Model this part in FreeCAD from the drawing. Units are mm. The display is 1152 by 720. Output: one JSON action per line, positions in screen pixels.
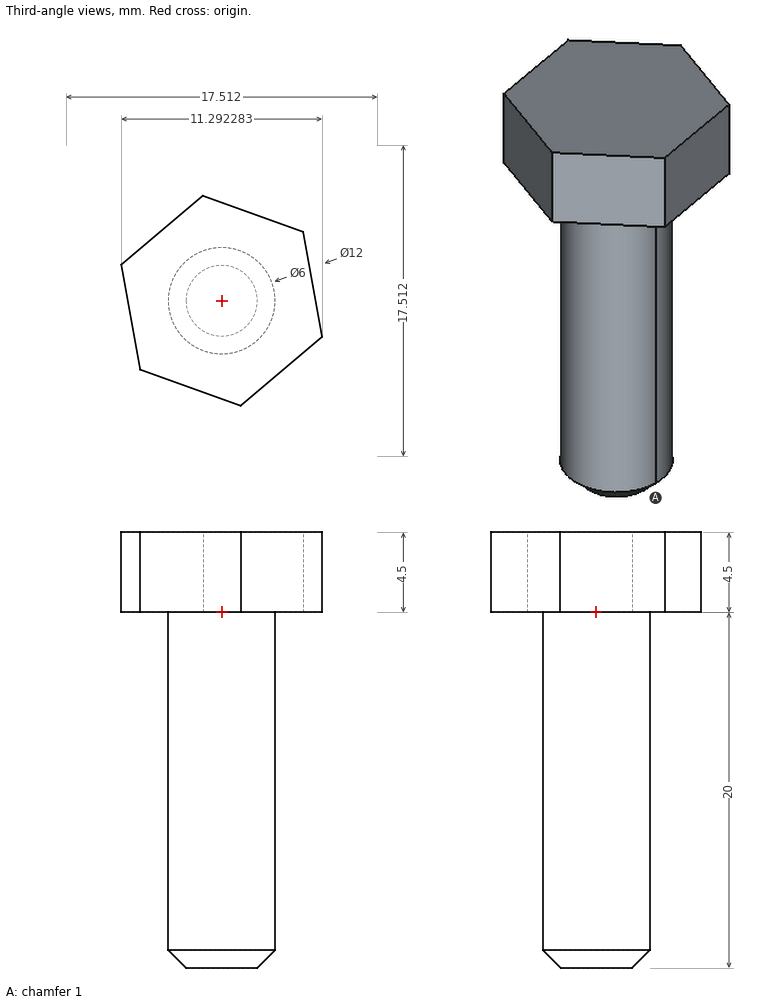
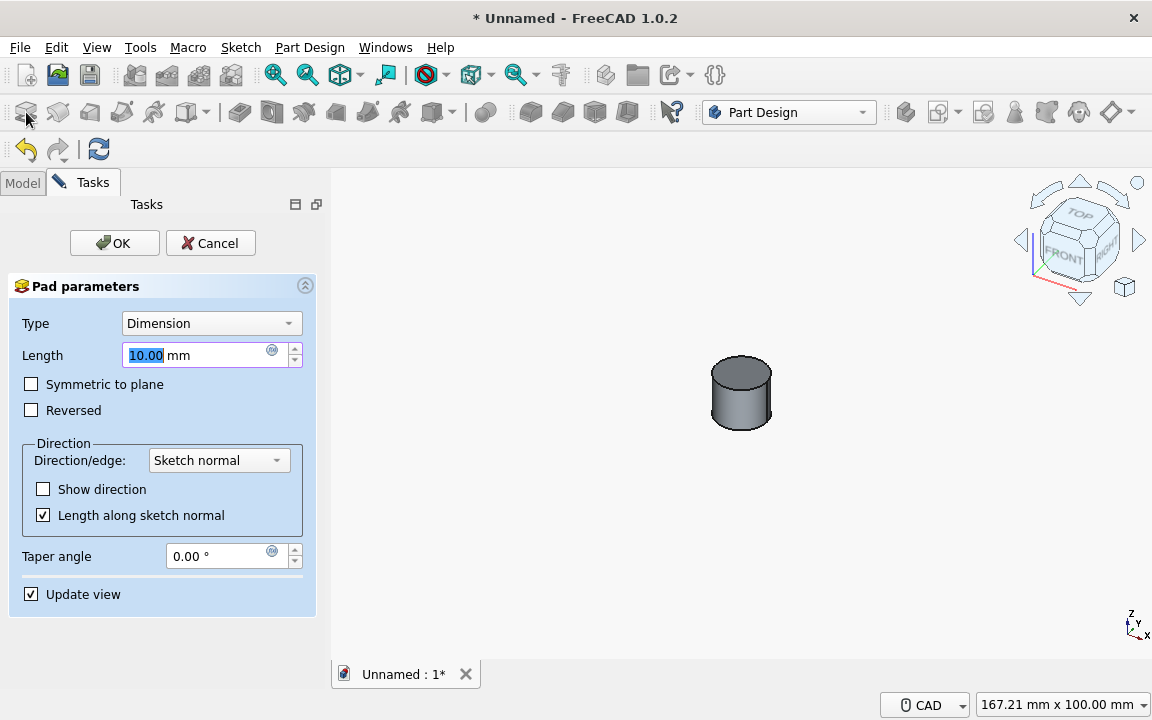
{"action": "type", "text": "4.5"}
{"action": "key", "text": "Tab"}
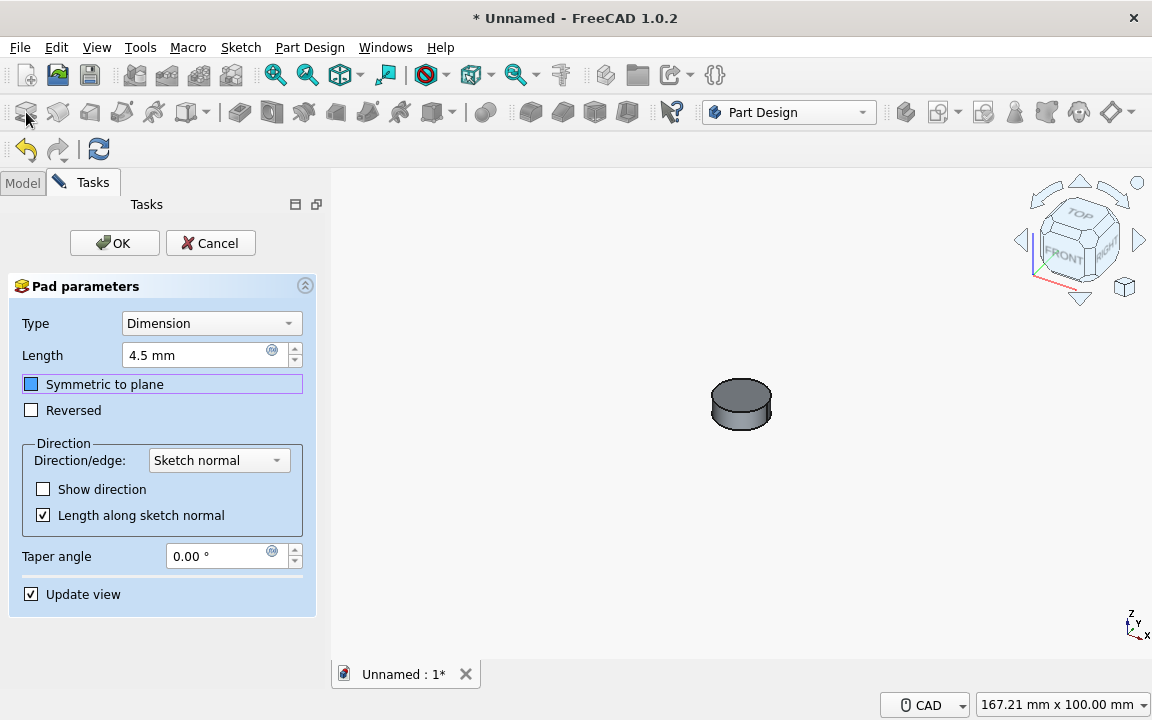
{"action": "left_click", "coordinate": [115, 243]}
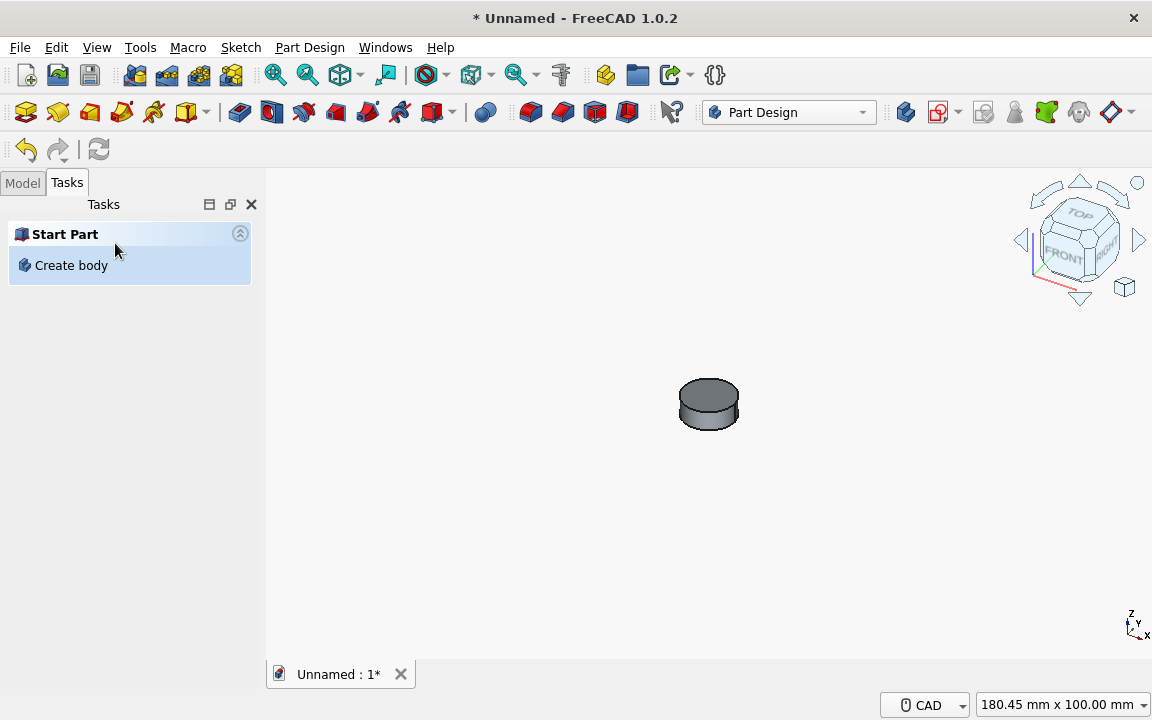
{"action": "key", "text": "v f"}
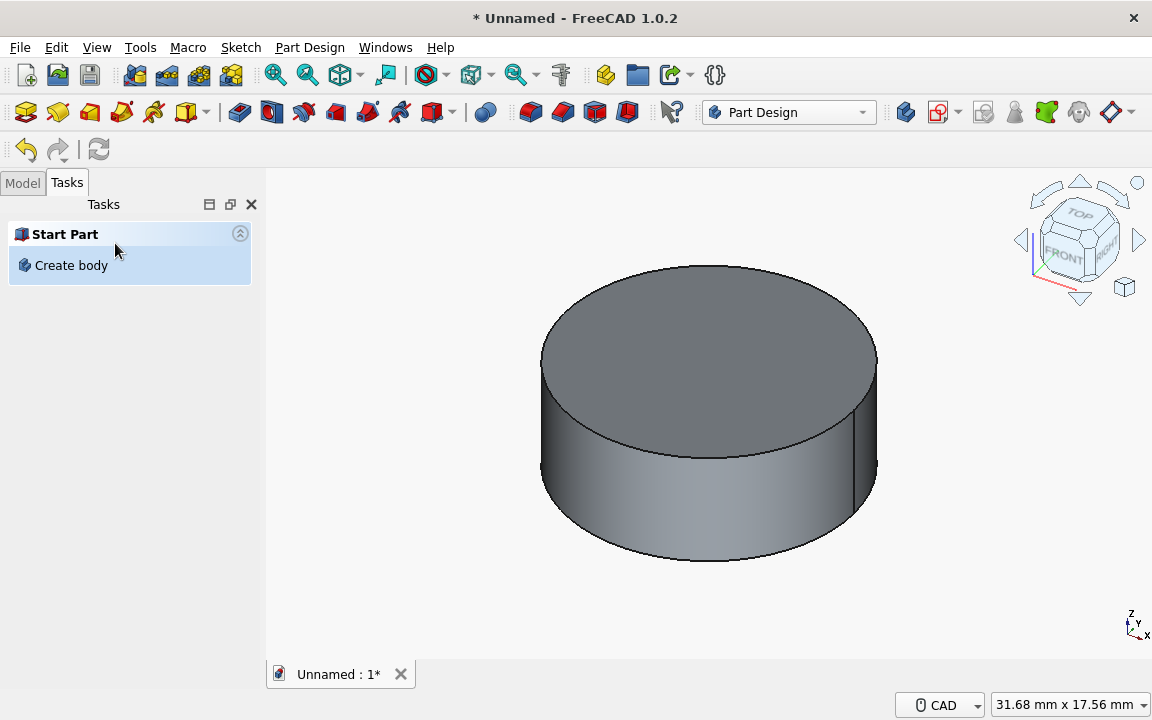
{"action": "key", "text": "5"}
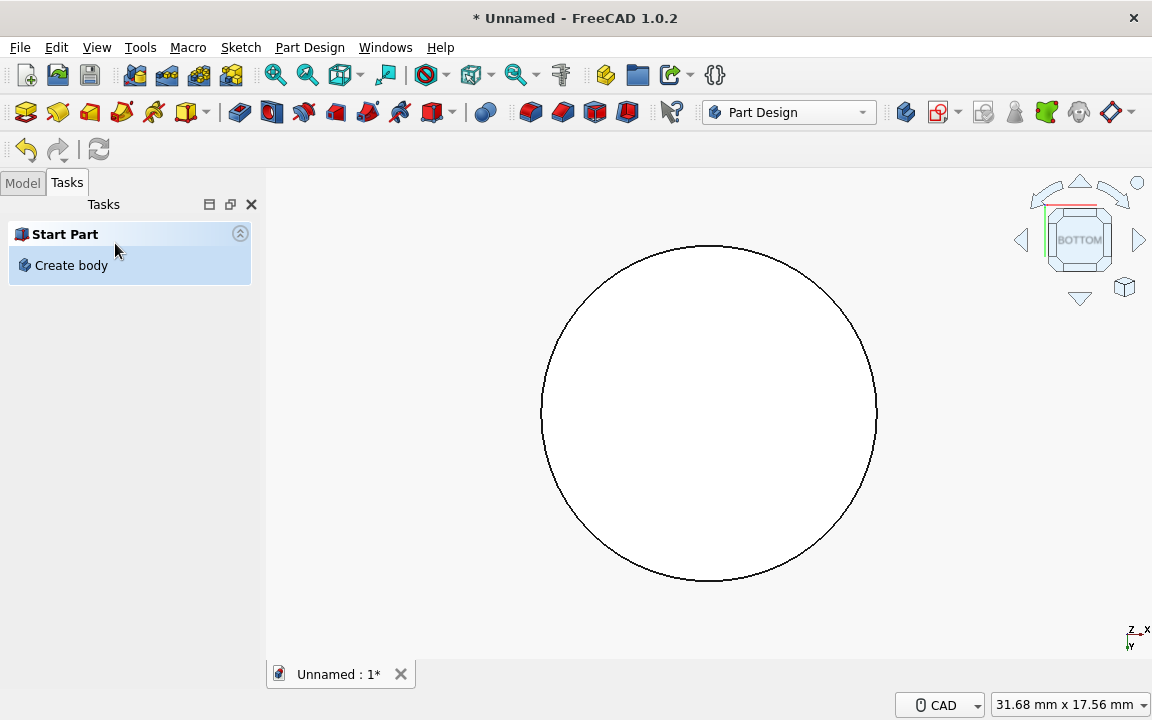
{"action": "left_click", "coordinate": [709, 412]}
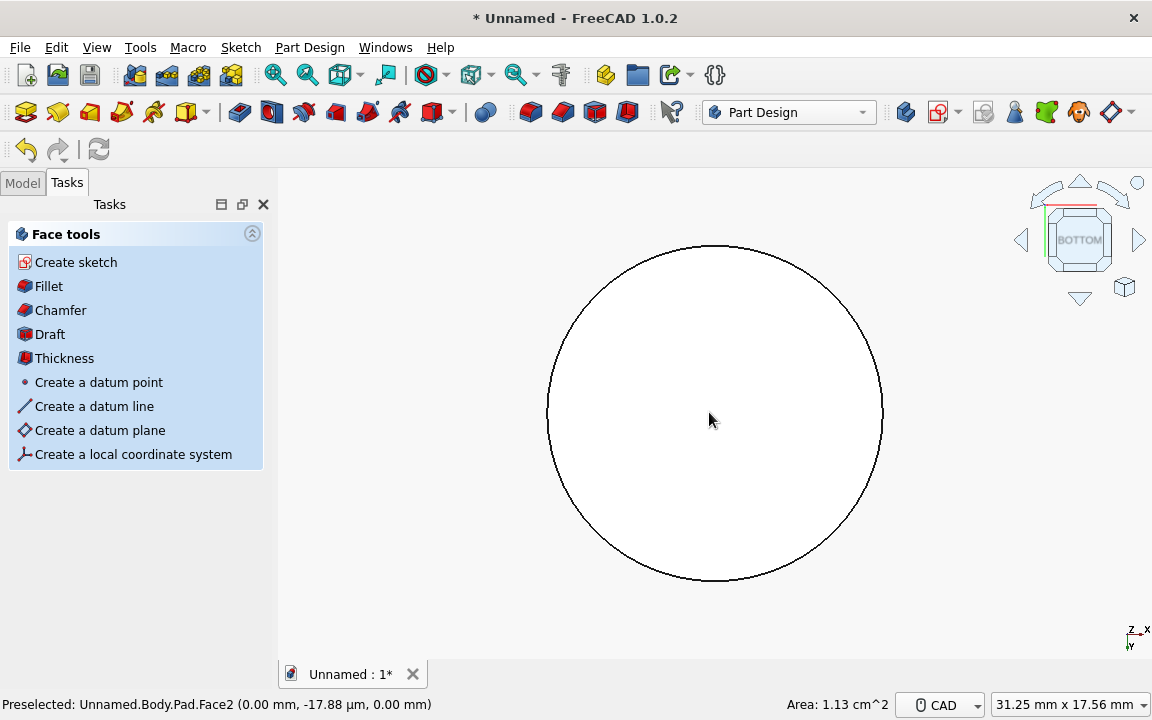
{"action": "left_click", "coordinate": [938, 112]}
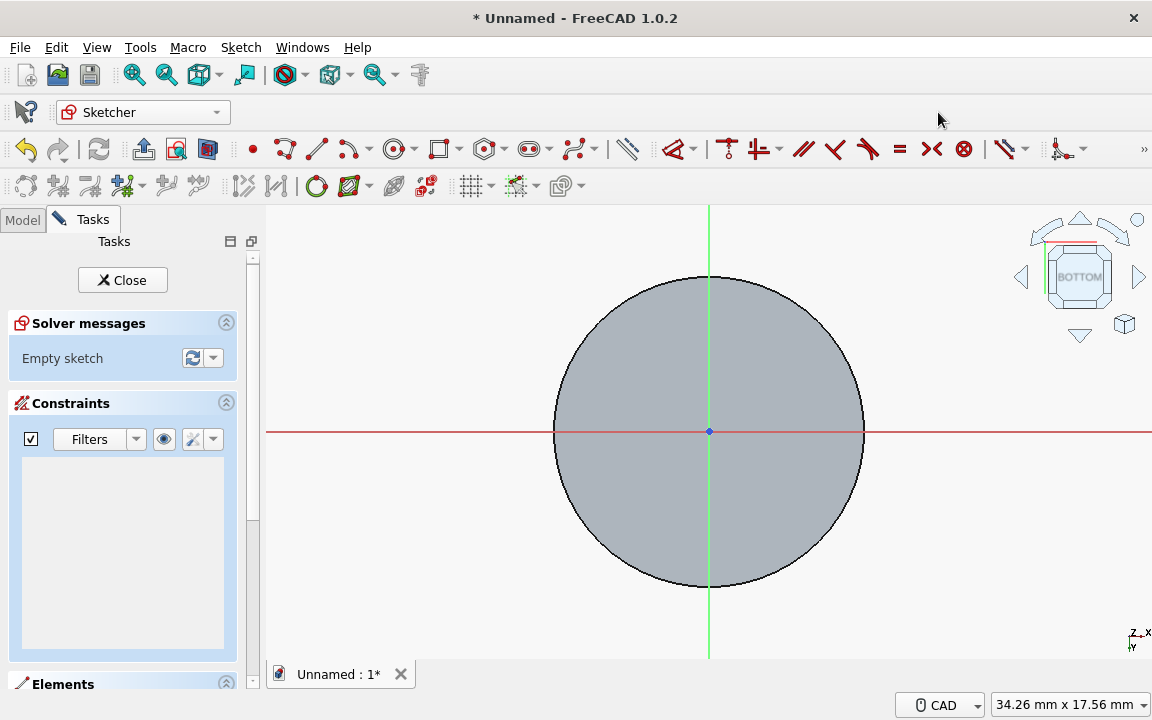
{"action": "scroll", "coordinate": [501, 432], "scroll_direction": "down", "scroll_amount": 2}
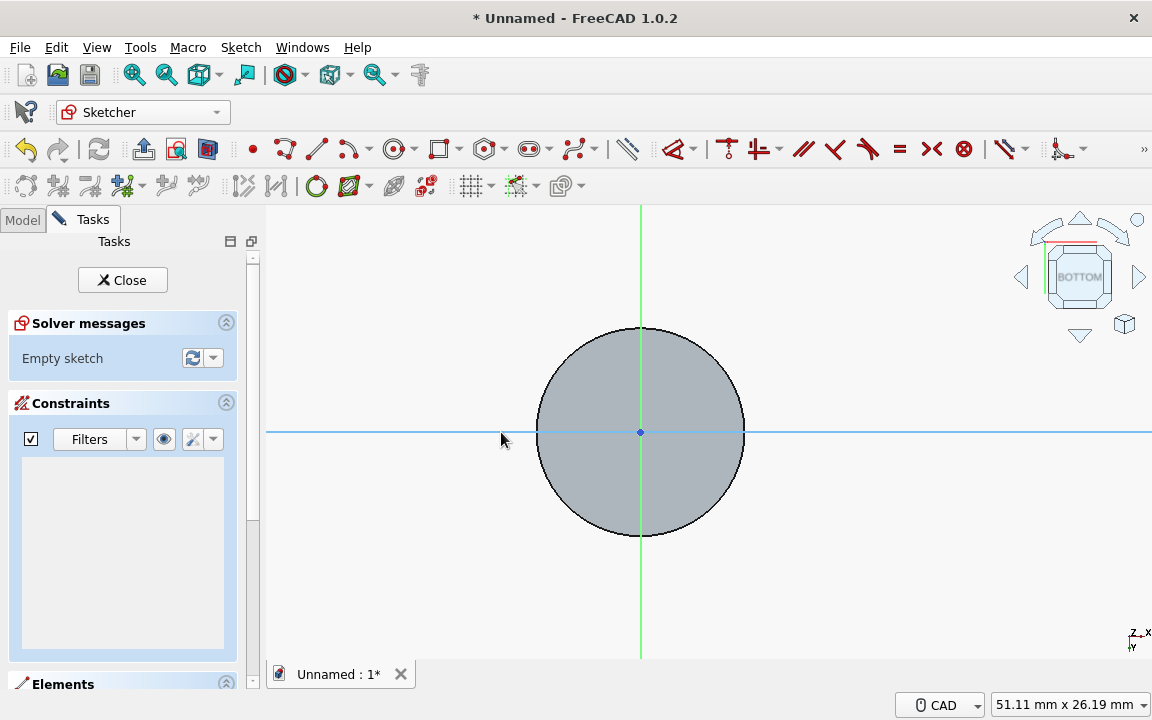
{"action": "left_click", "coordinate": [462, 150]}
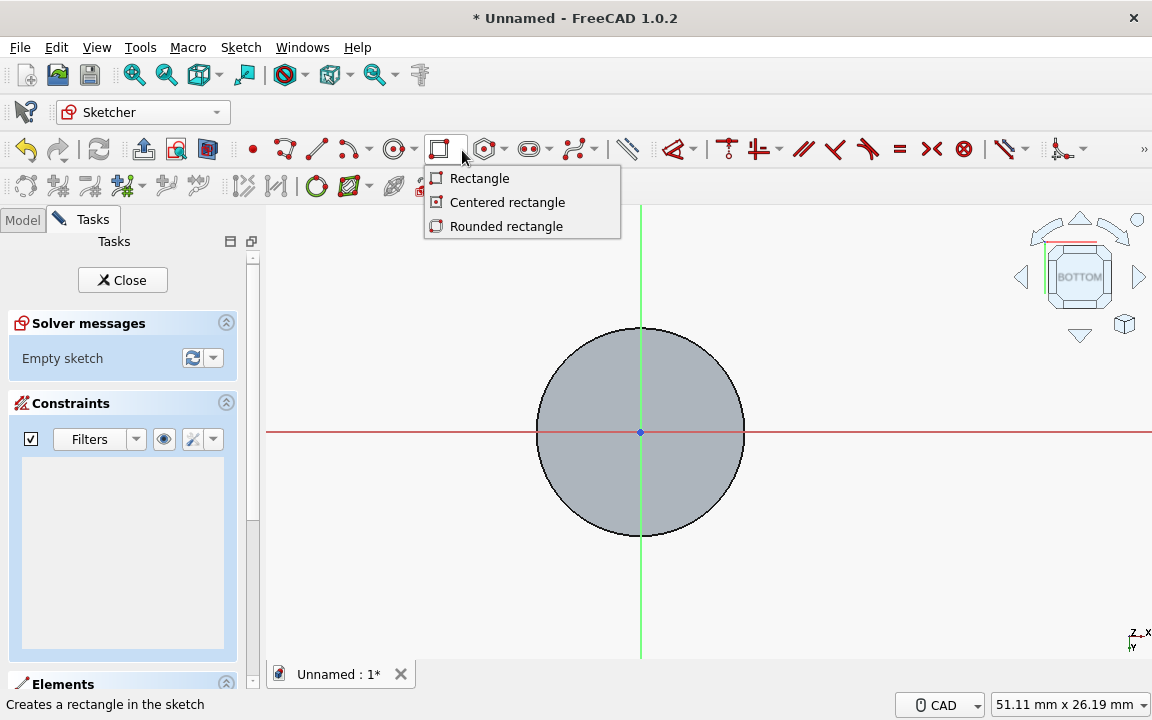
{"action": "left_click", "coordinate": [522, 202]}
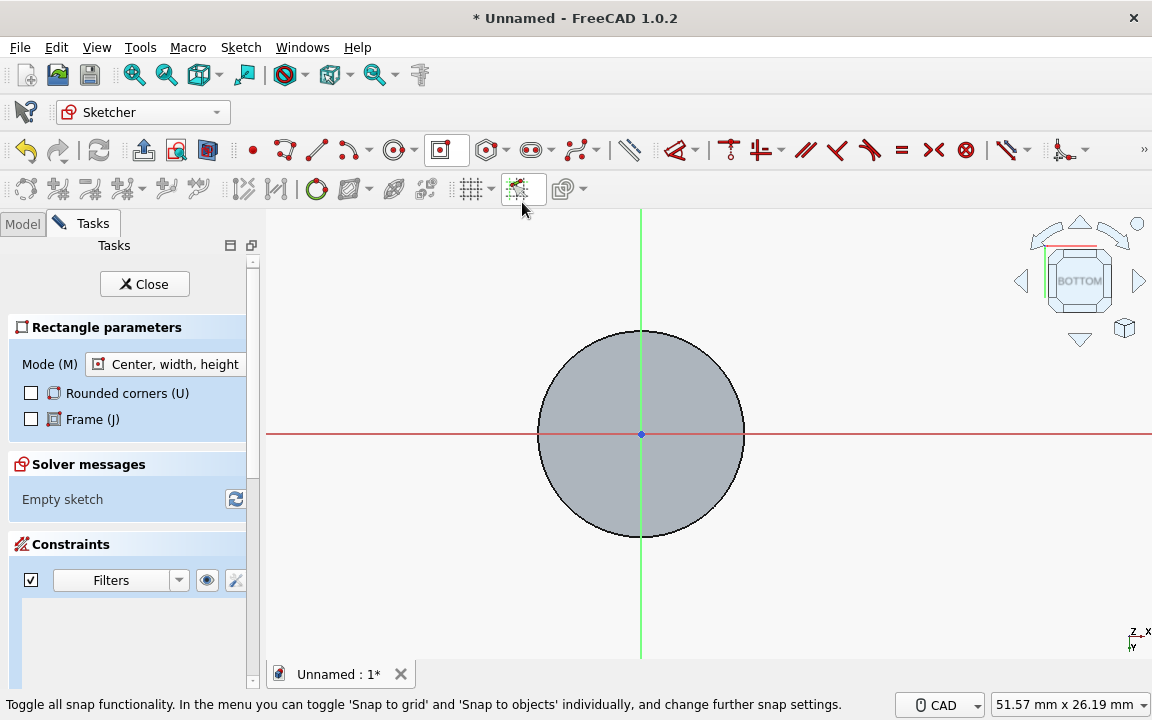
{"action": "left_click", "coordinate": [641, 434]}
{"action": "left_click", "coordinate": [792, 284]}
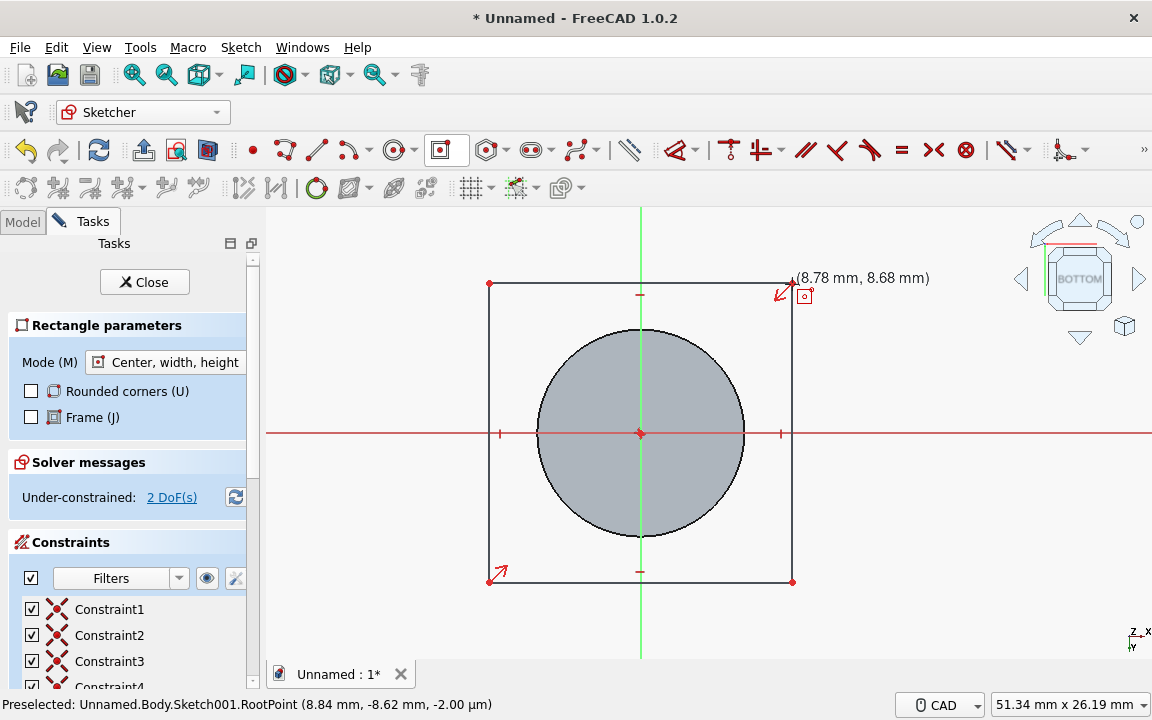
{"action": "key", "text": "g p 6"}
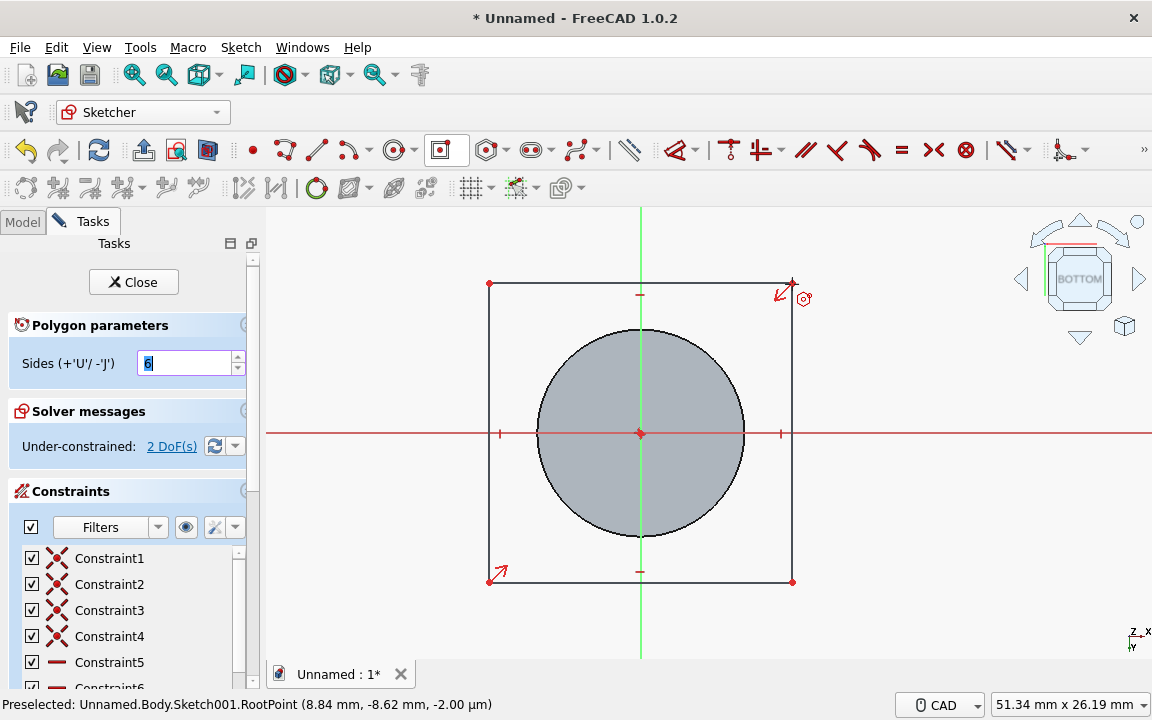
{"action": "left_click", "coordinate": [641, 433]}